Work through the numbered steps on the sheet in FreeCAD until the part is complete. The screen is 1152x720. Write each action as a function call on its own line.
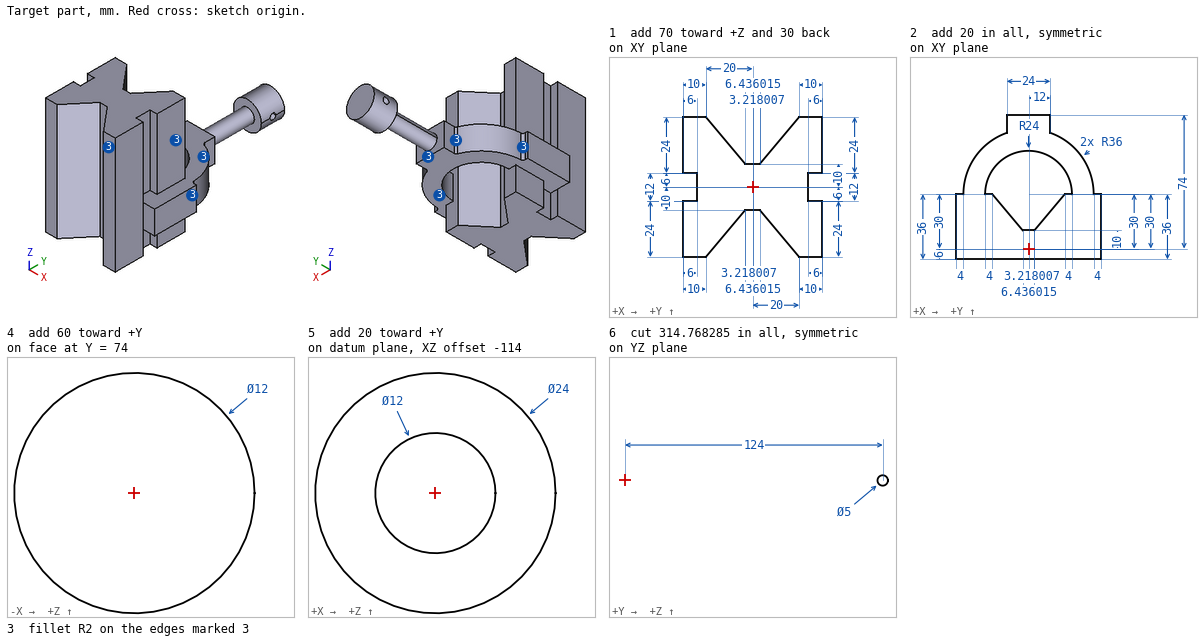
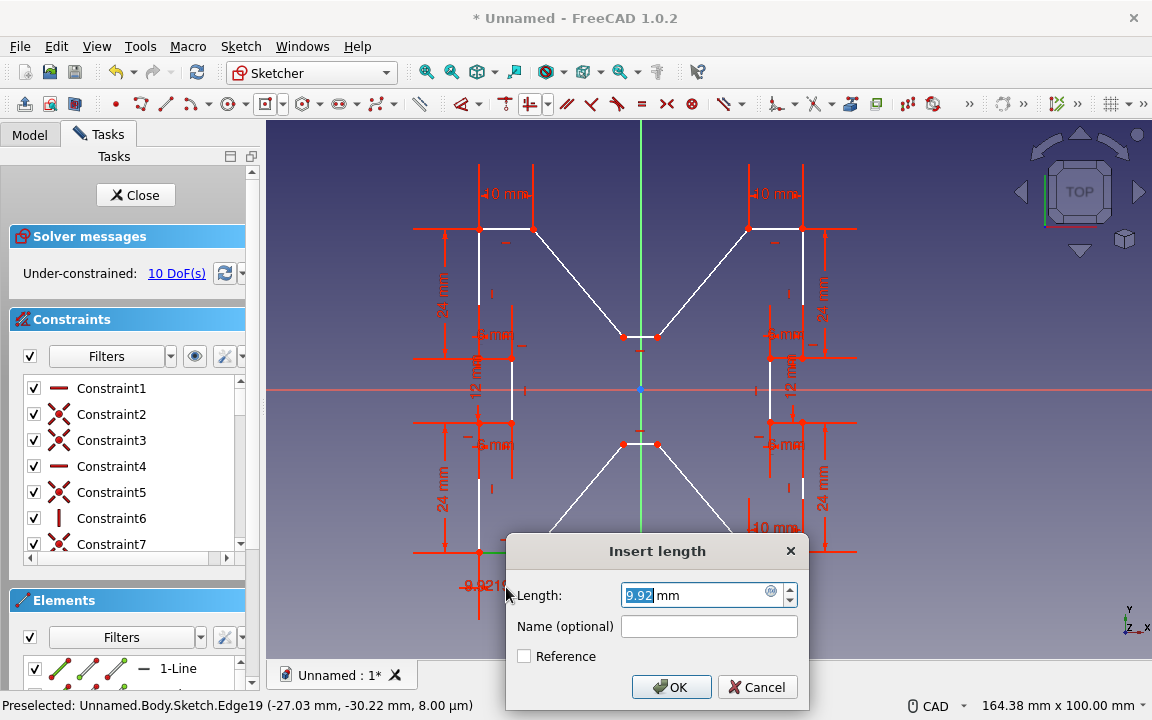
text(10)
key(Return)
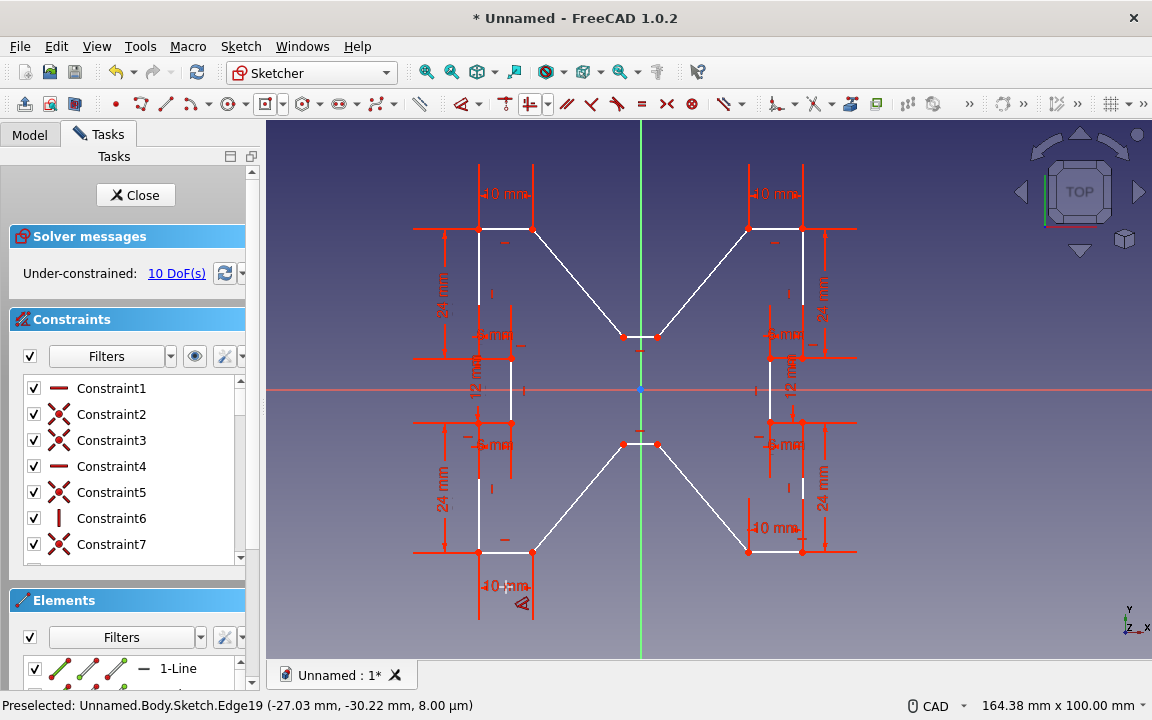
scroll(803, 423, up, 2)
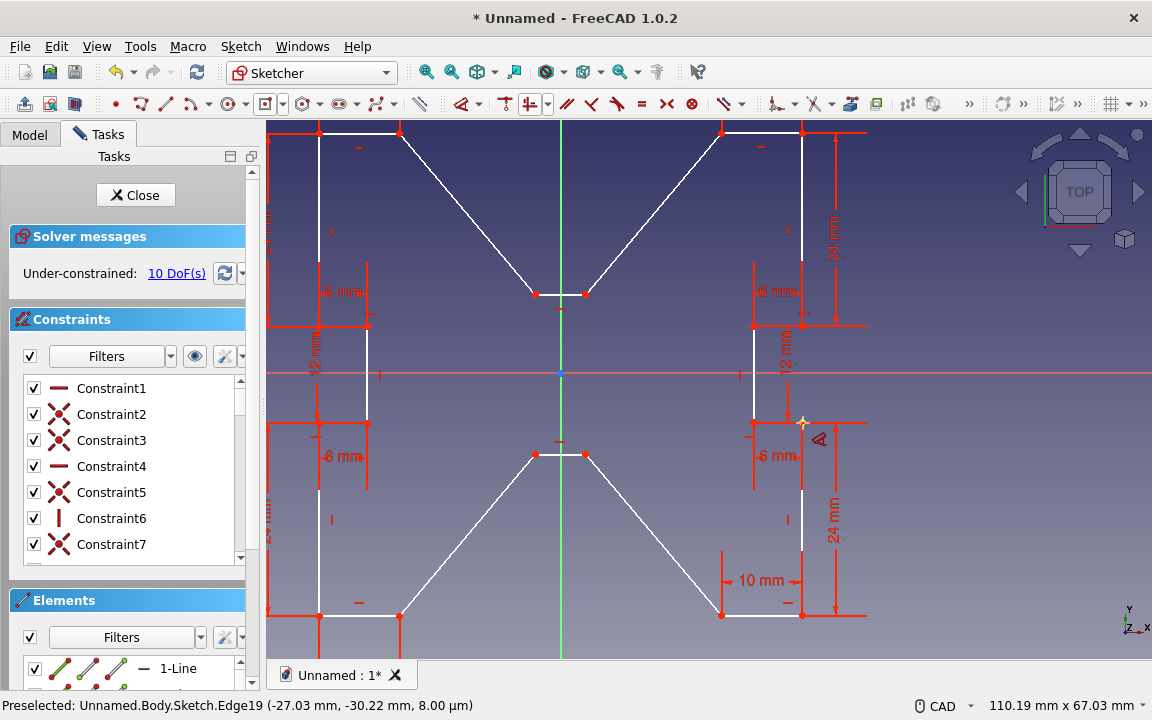
click(802, 423)
click(836, 398)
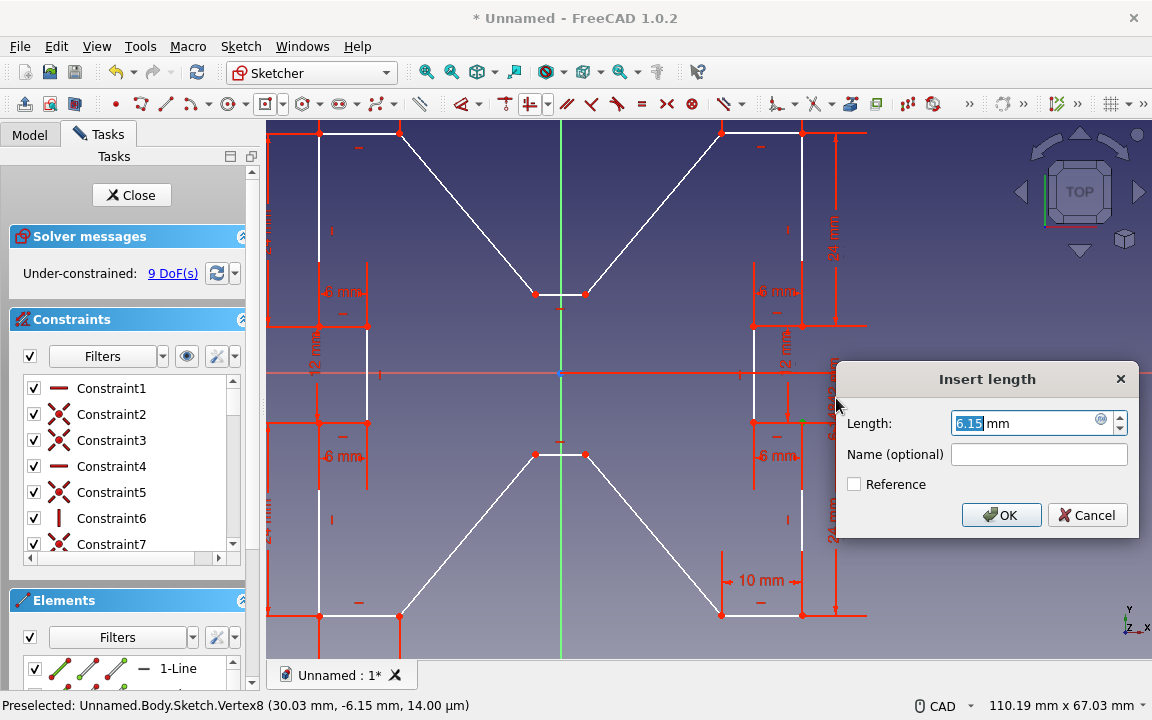
text(6)
key(Return)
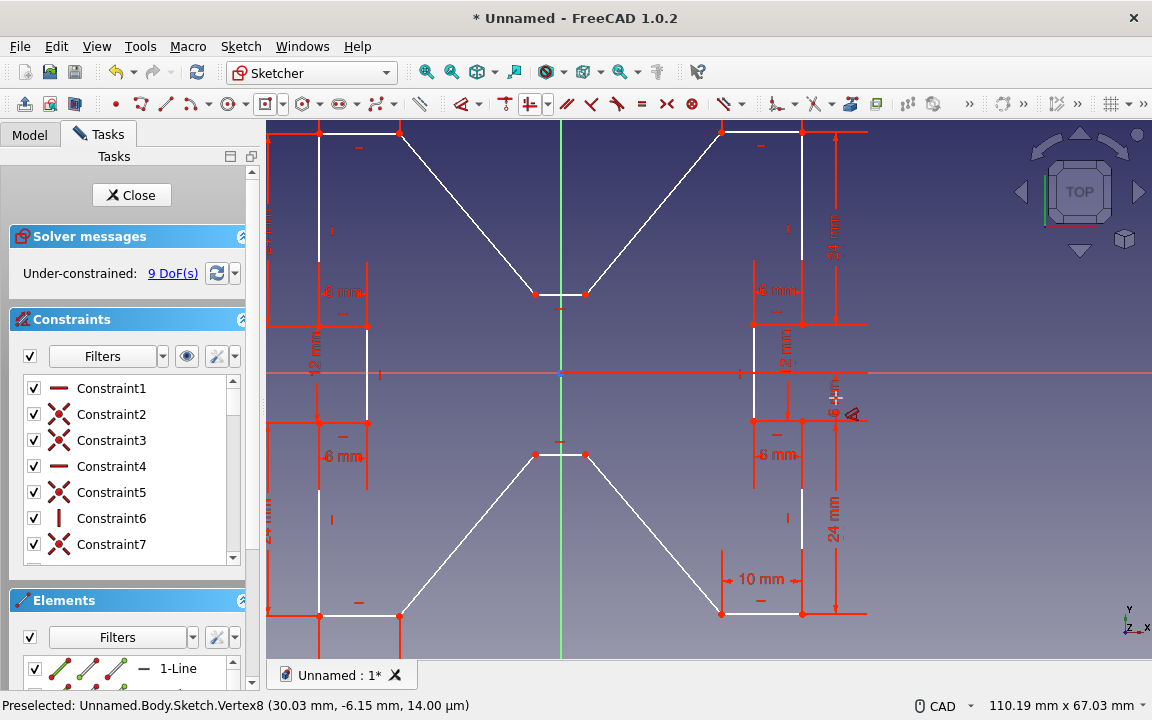
click(319, 327)
click(595, 350)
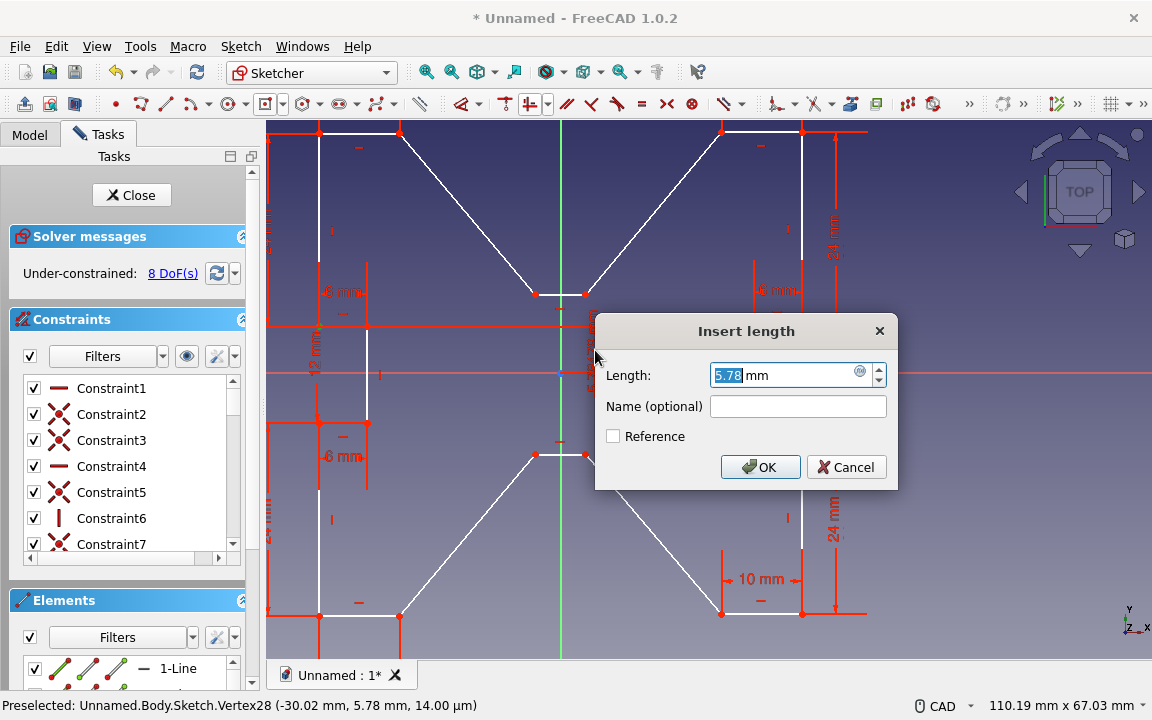
text(6)
key(Return)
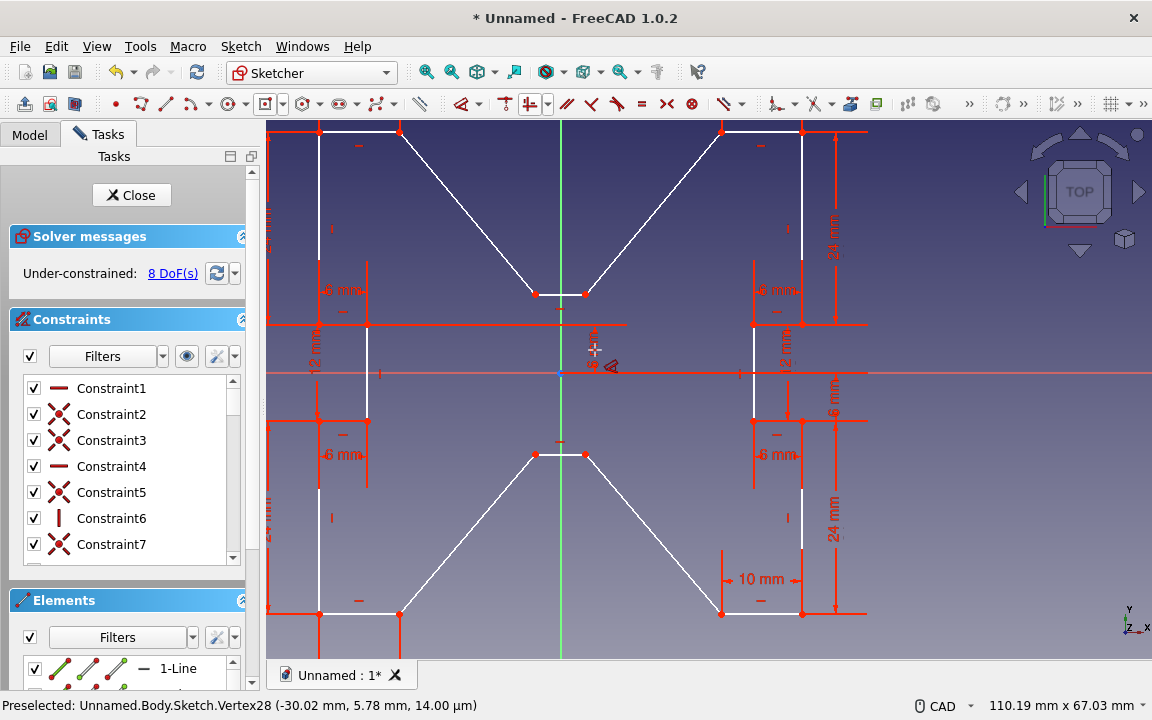
click(535, 455)
click(501, 414)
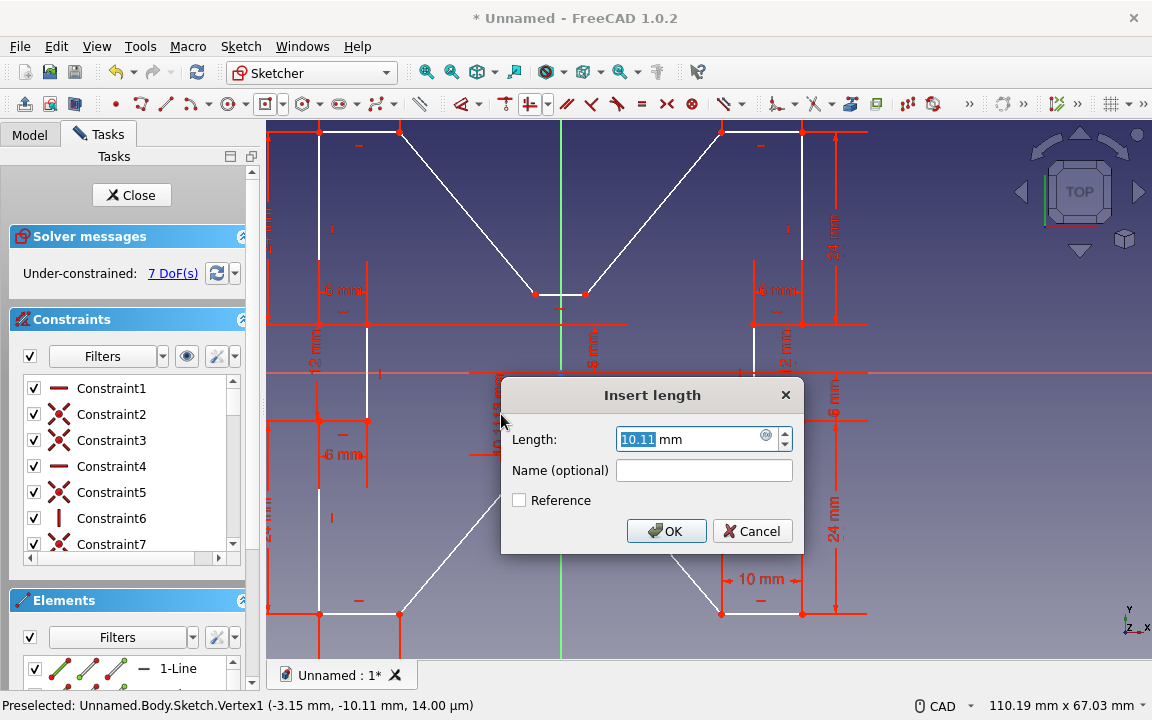
text(10)
key(Return)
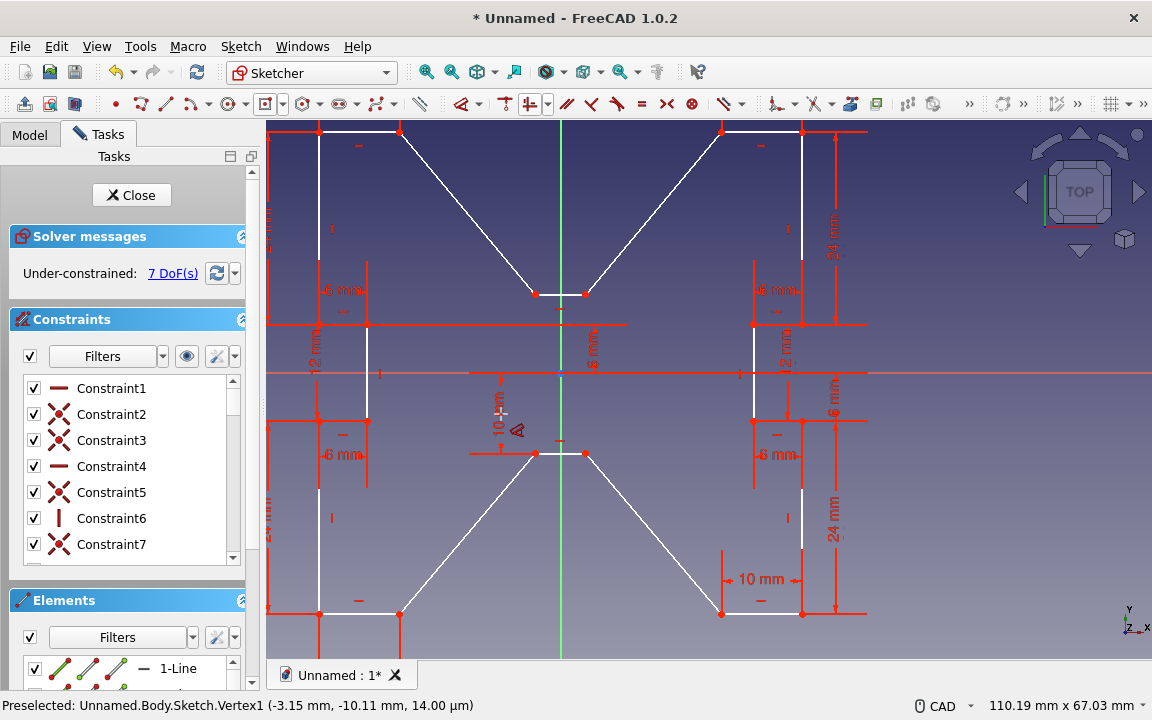
click(722, 614)
click(678, 339)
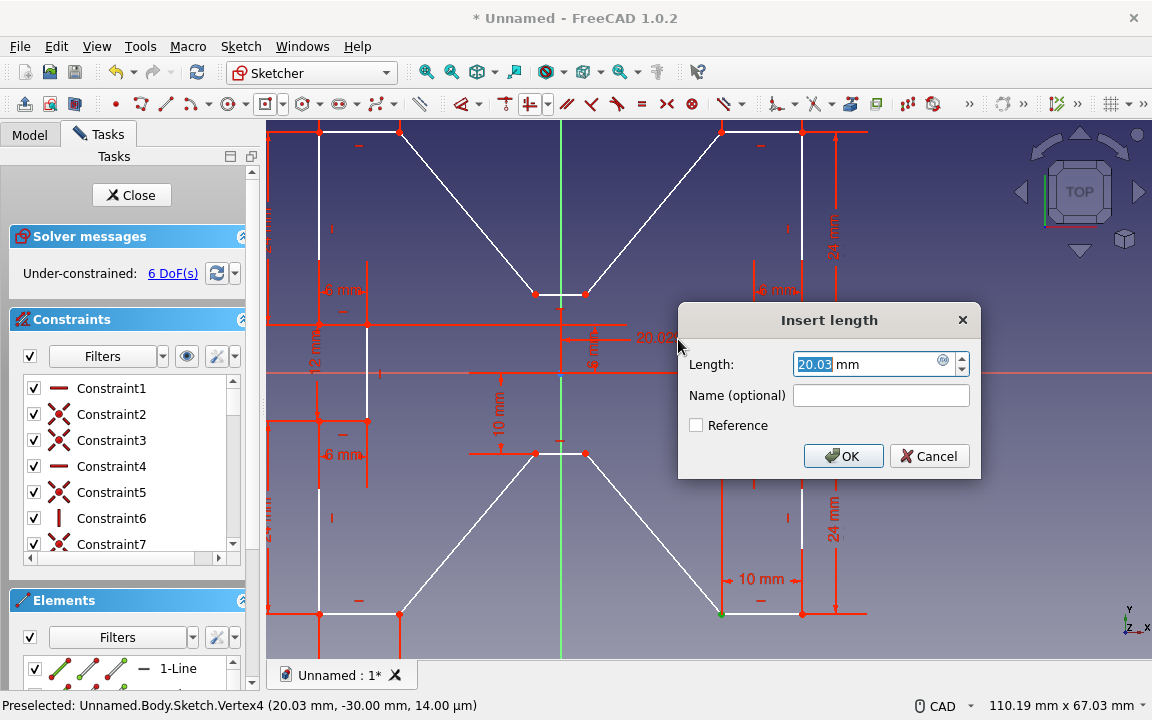
text(20)
key(Return)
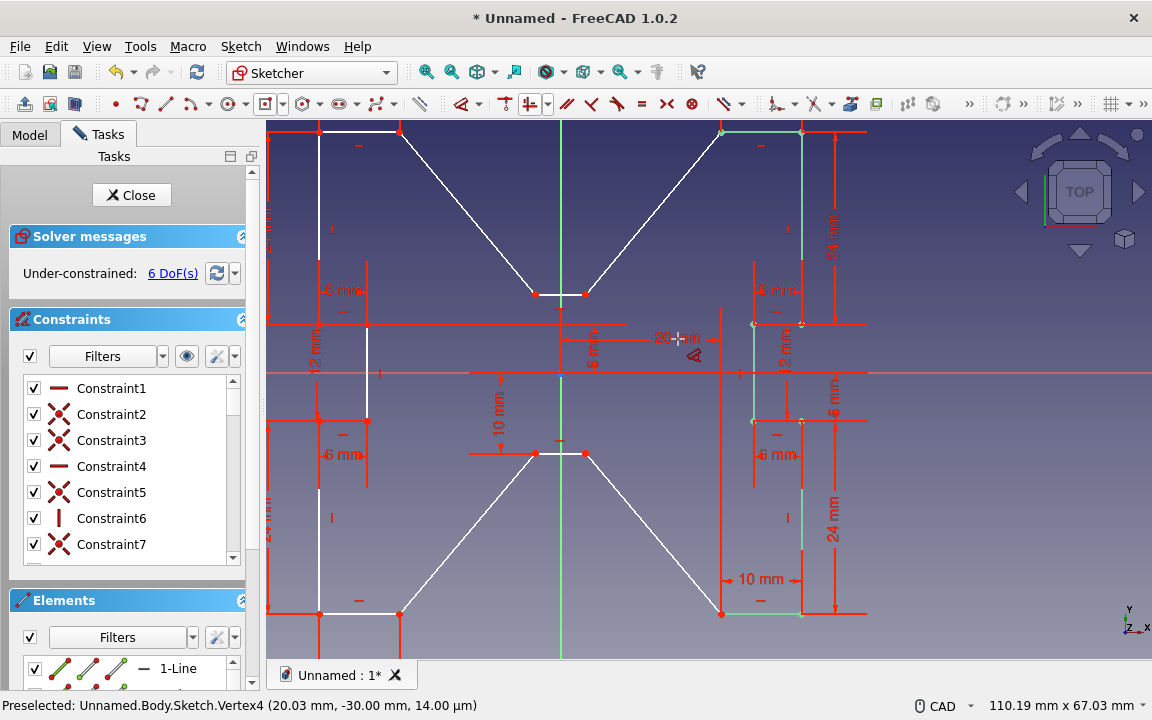
click(586, 295)
click(620, 316)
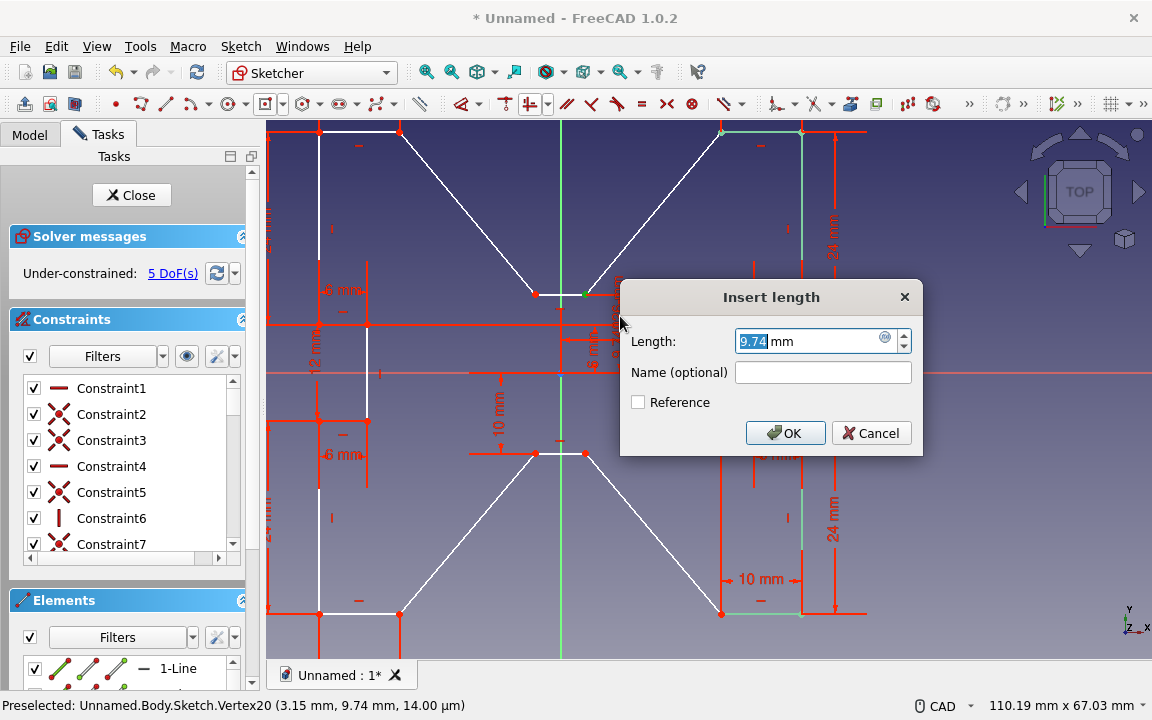
text(10)
key(Return)